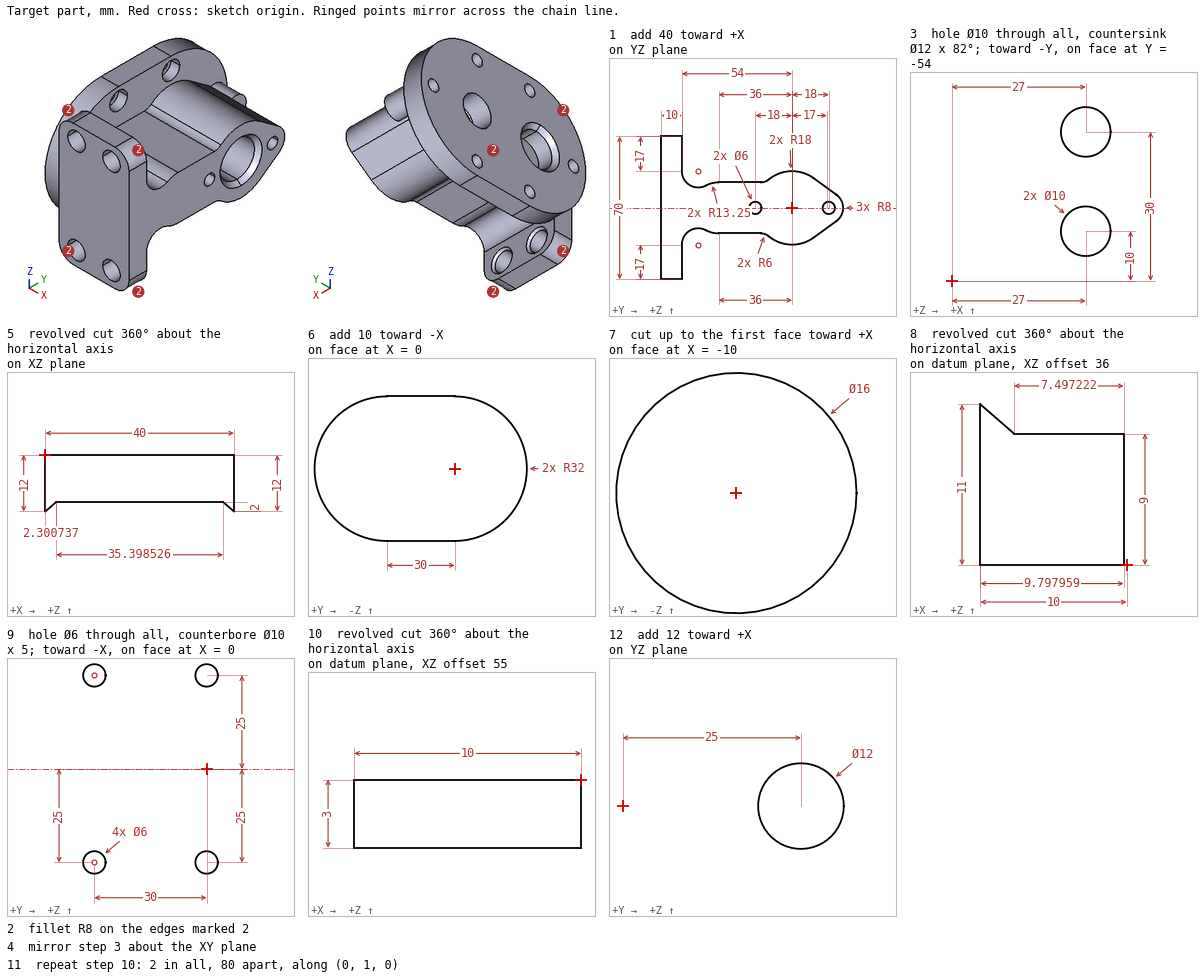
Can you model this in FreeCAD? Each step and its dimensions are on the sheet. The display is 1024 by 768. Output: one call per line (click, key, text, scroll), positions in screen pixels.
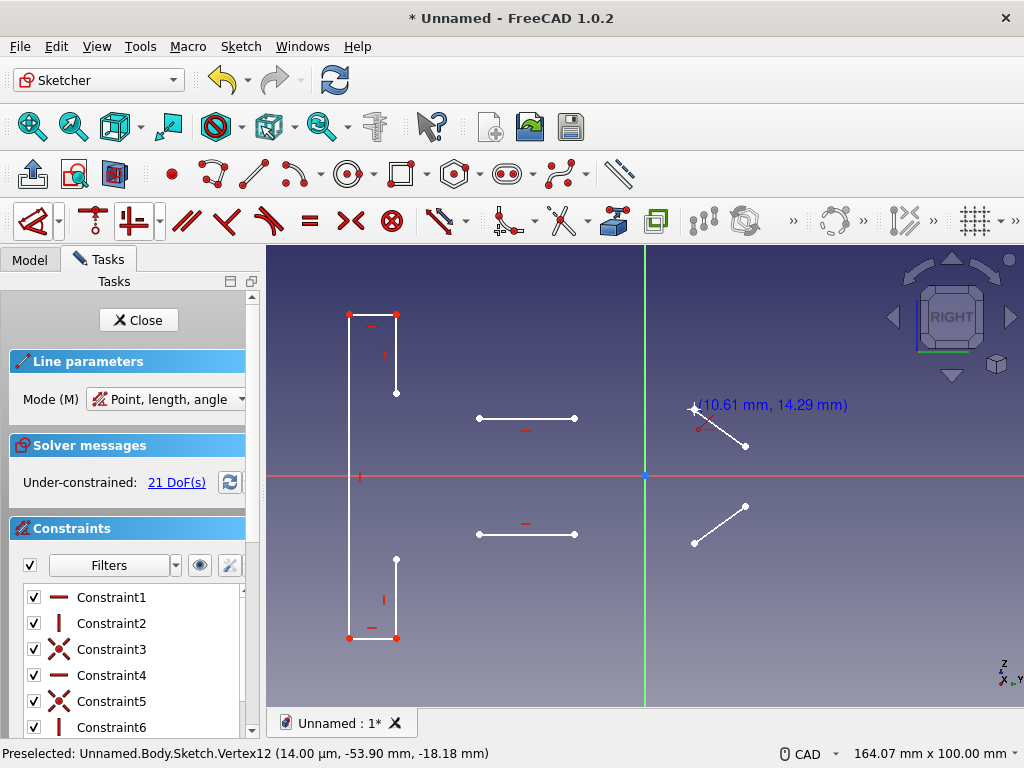
click(320, 174)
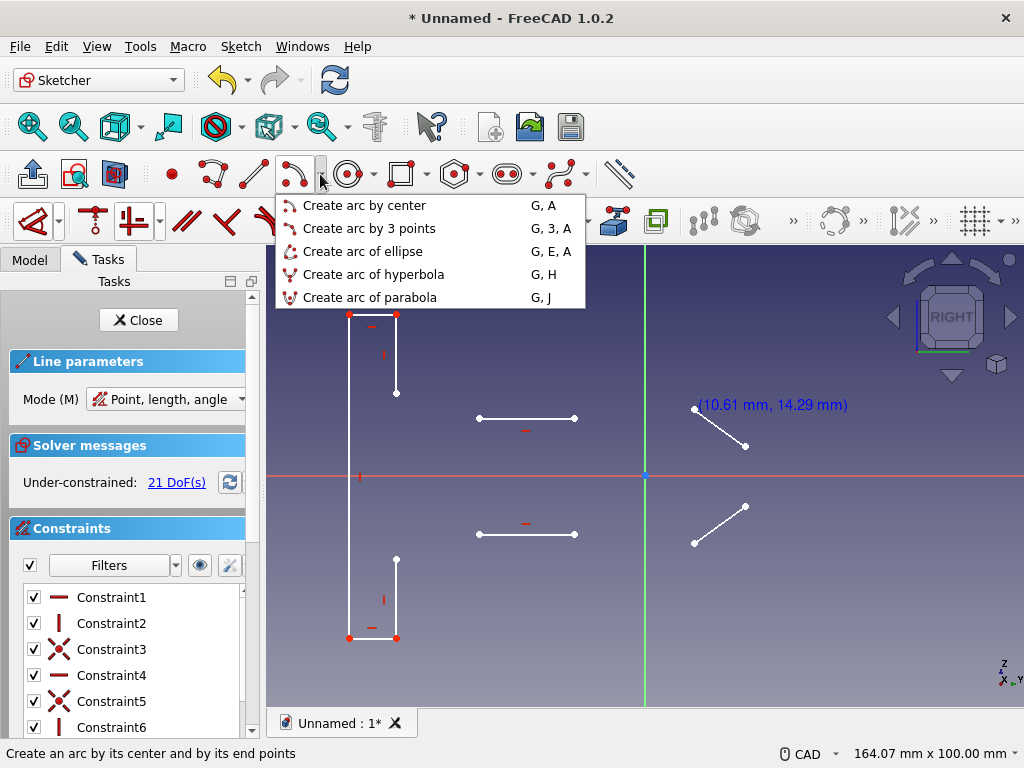
click(430, 228)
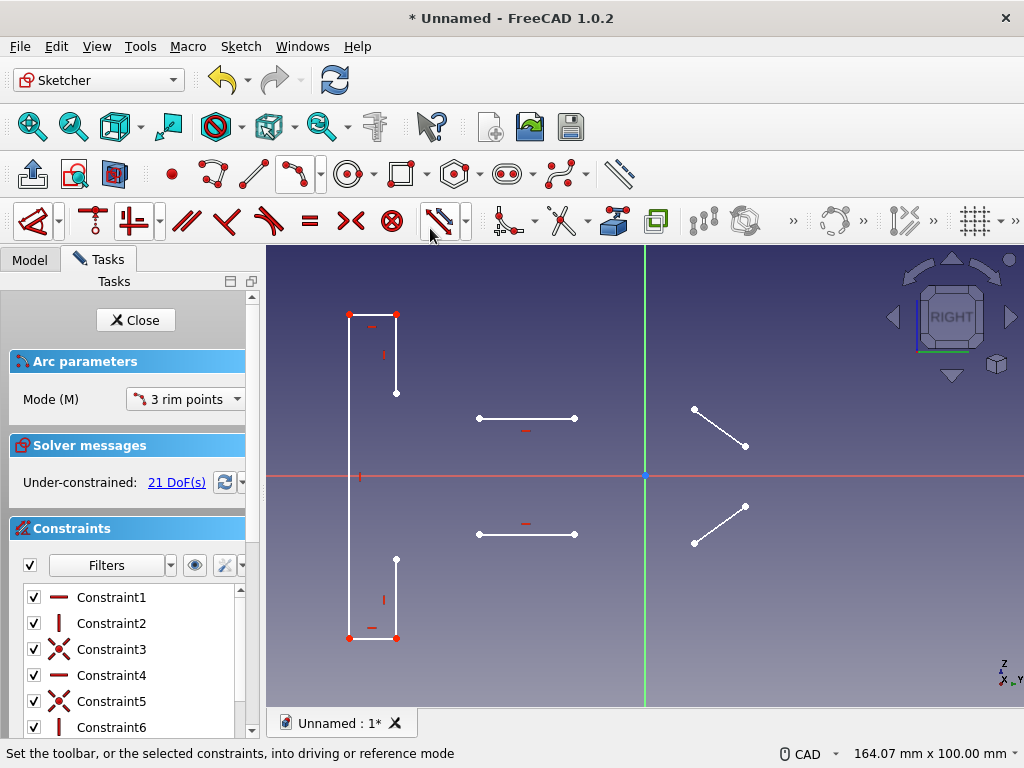
click(479, 419)
click(450, 425)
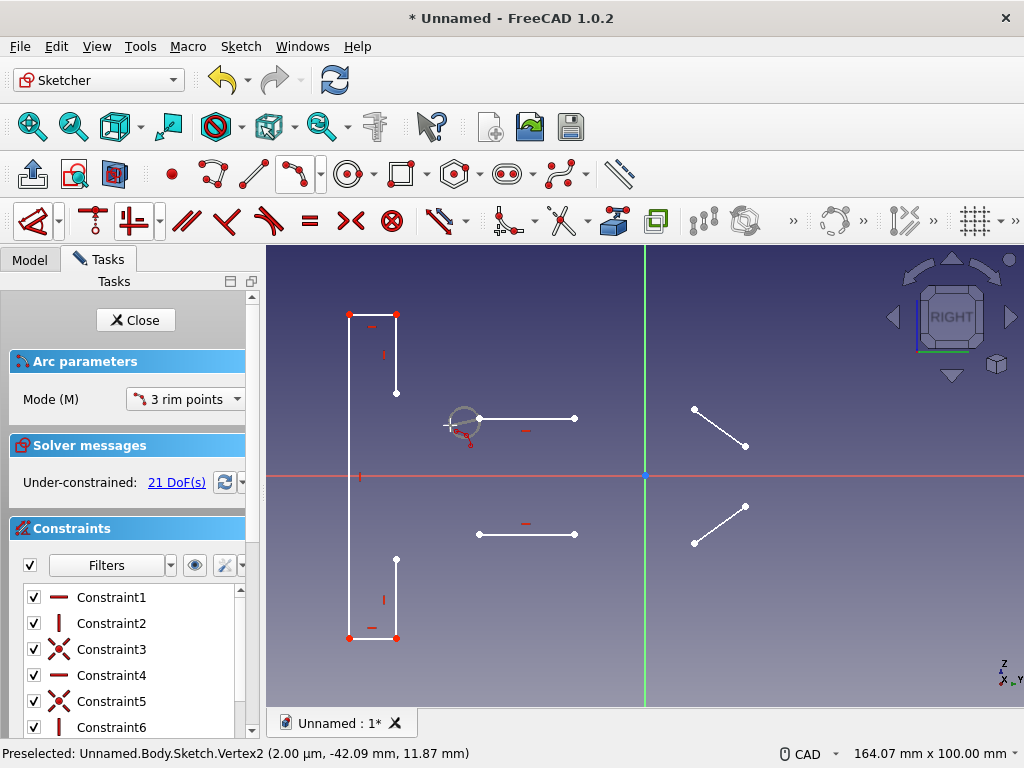
scroll(464, 420, up, 11)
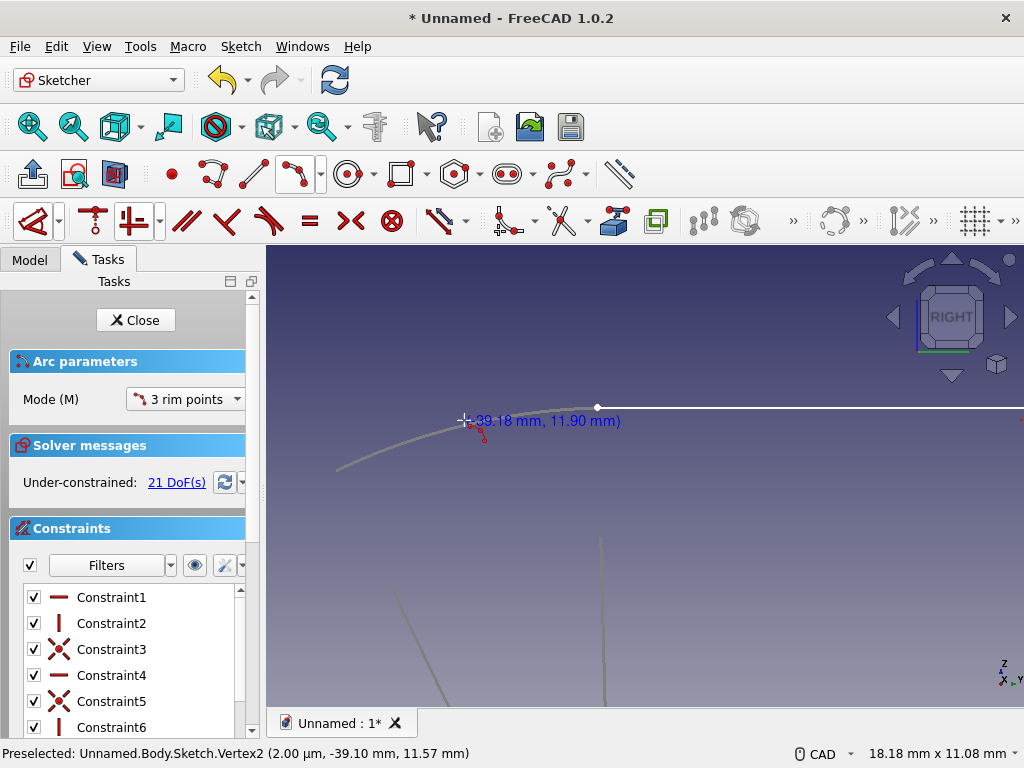
click(460, 418)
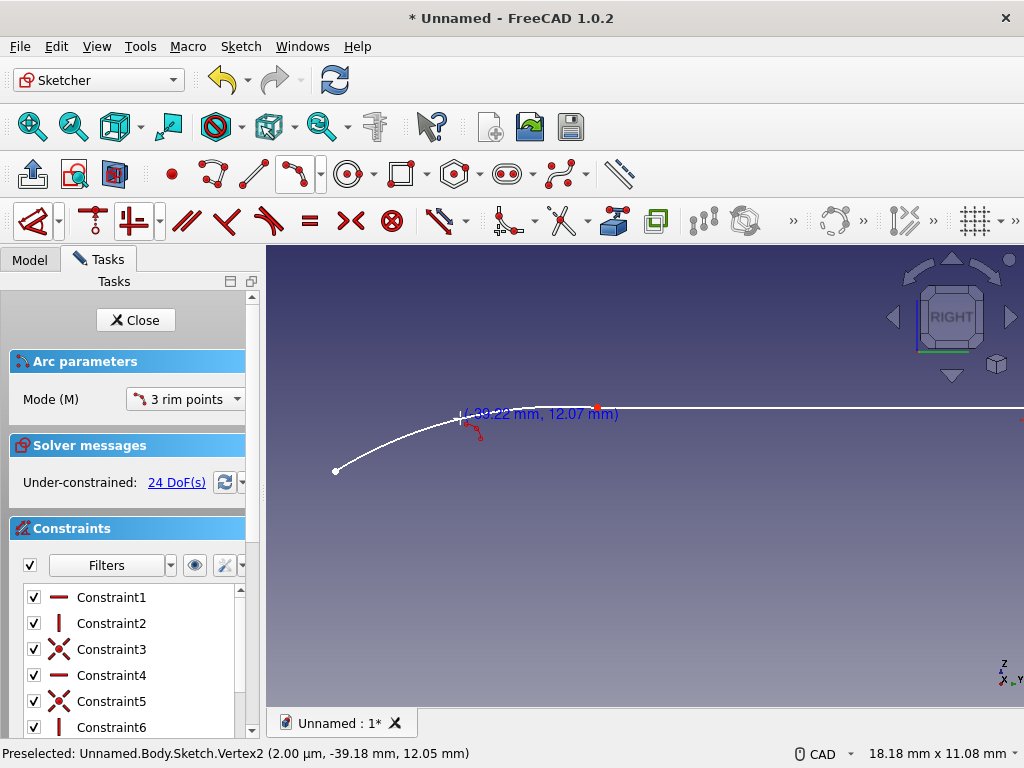
scroll(506, 431, down, 12)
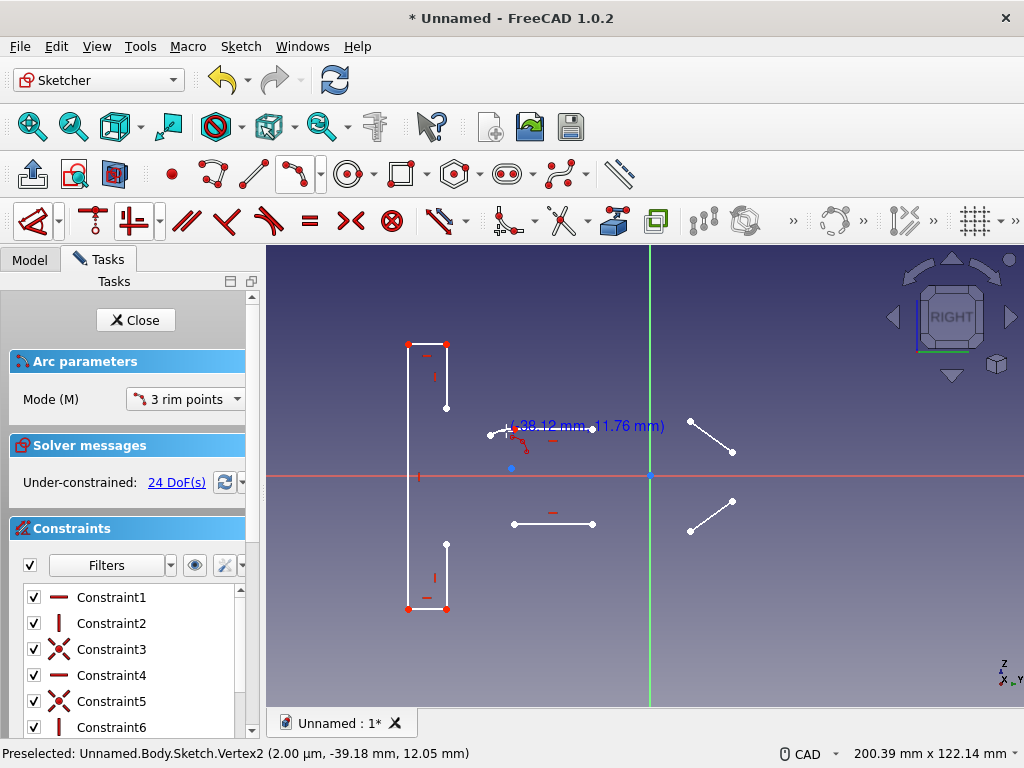
click(491, 435)
click(447, 409)
click(461, 434)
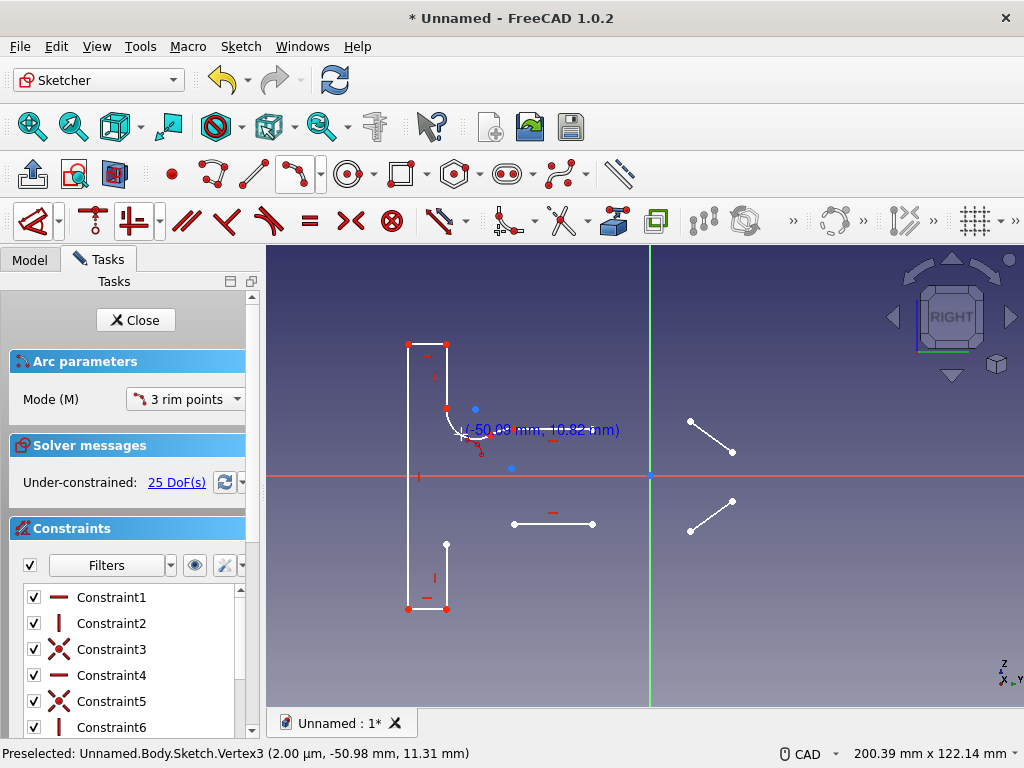
click(447, 545)
click(491, 517)
click(461, 518)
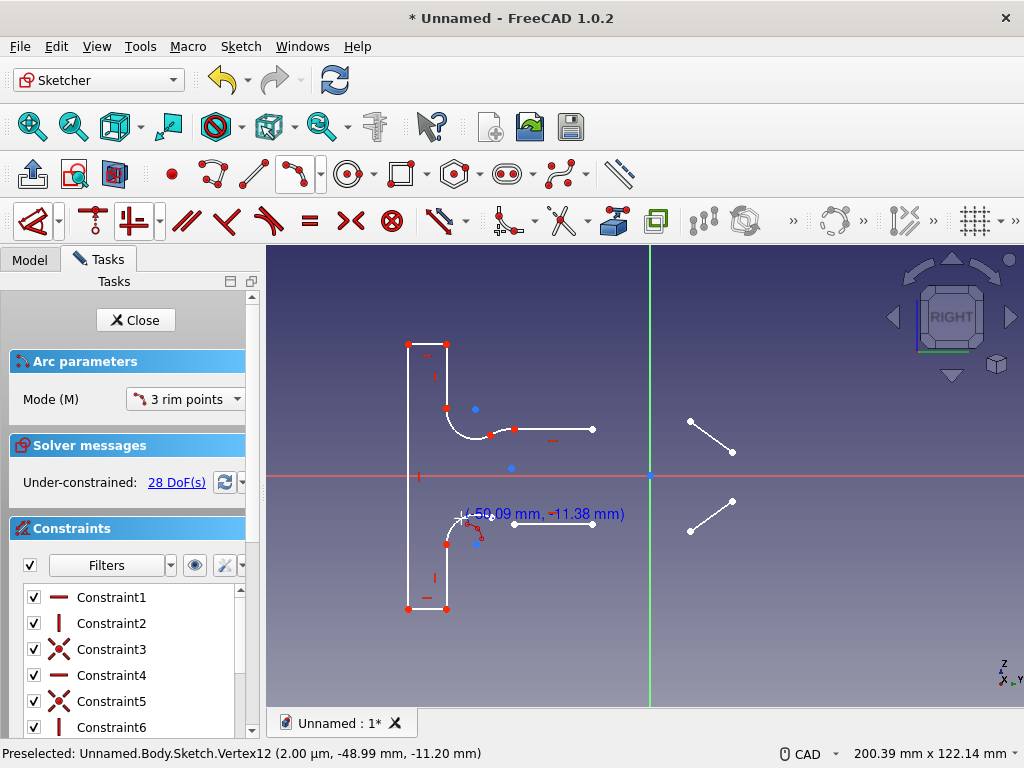
click(491, 518)
click(515, 524)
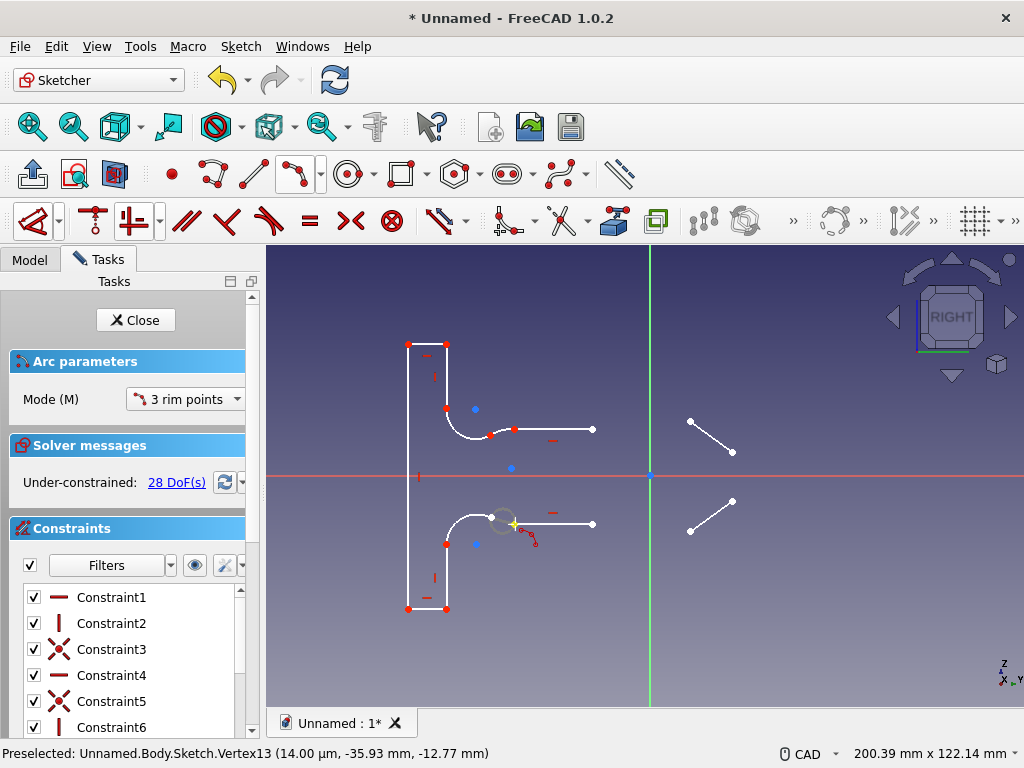
scroll(502, 522, up, 12)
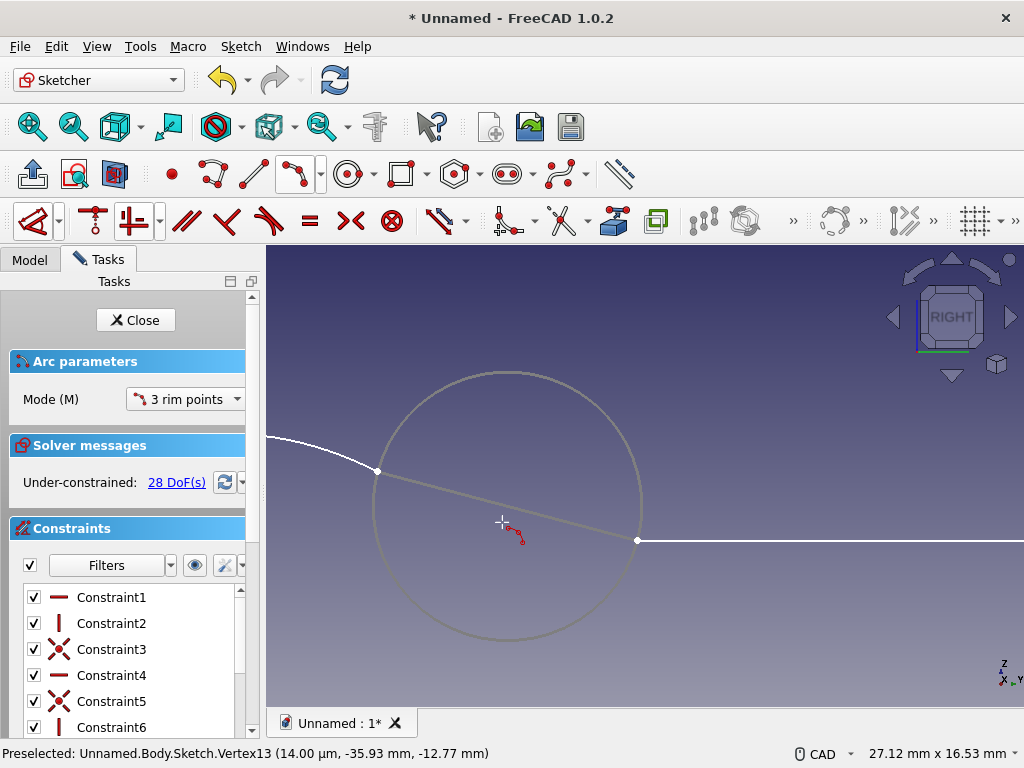
click(501, 513)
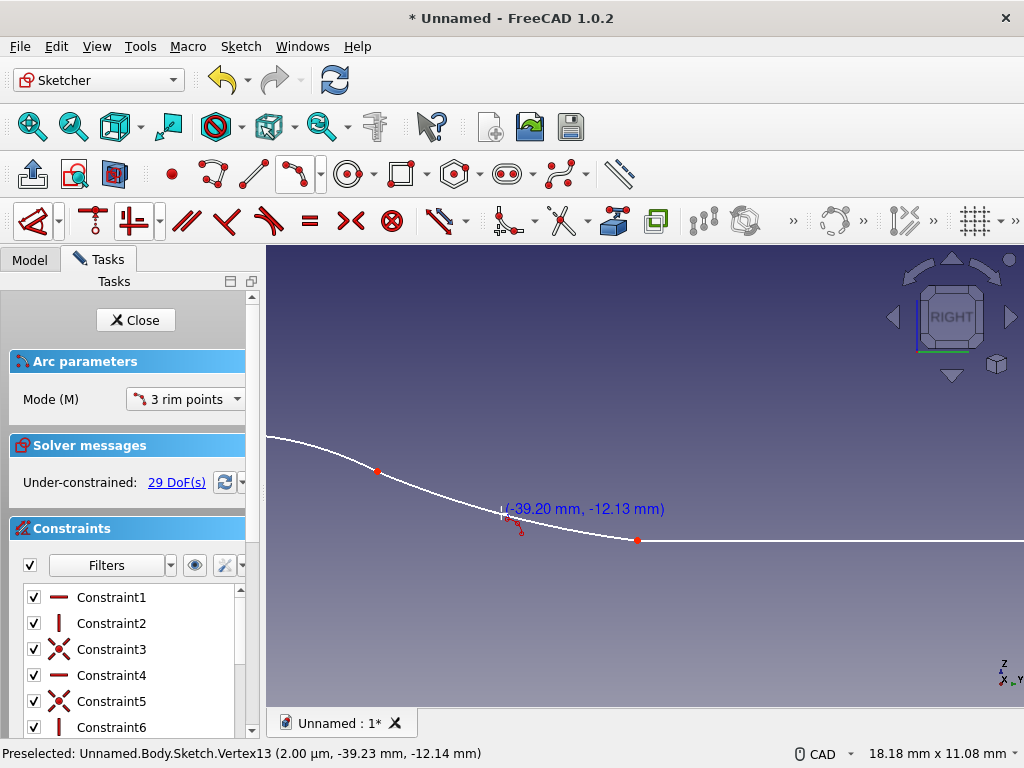
scroll(502, 523, down, 12)